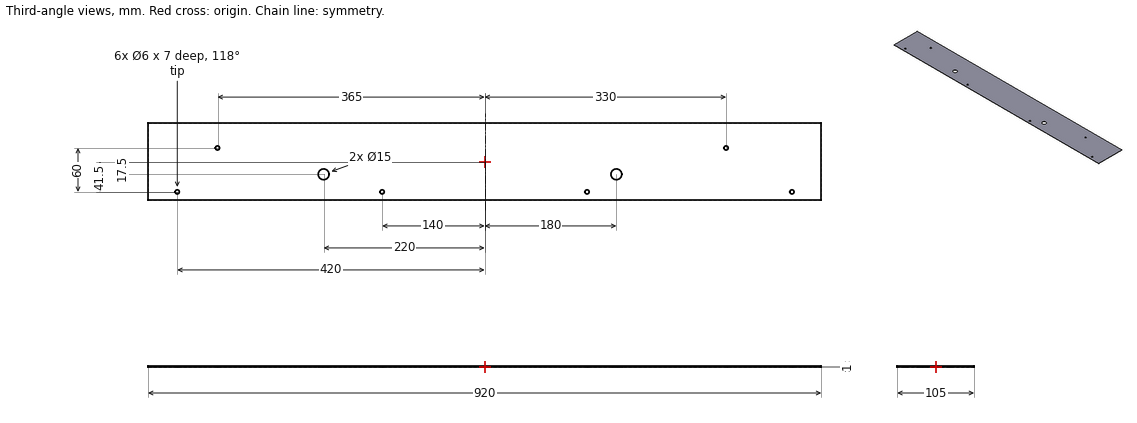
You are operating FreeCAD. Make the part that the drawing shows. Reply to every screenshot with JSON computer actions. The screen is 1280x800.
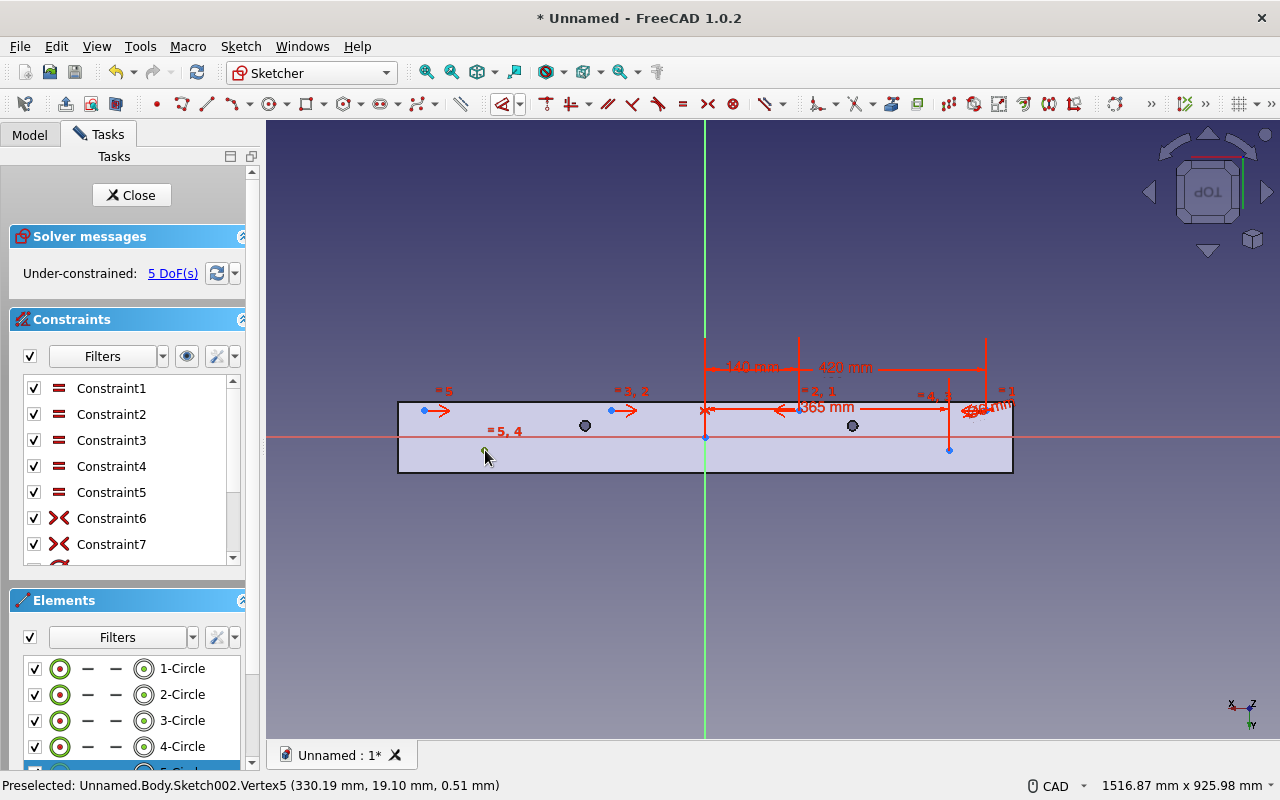
{"action": "left_click", "coordinate": [520, 104]}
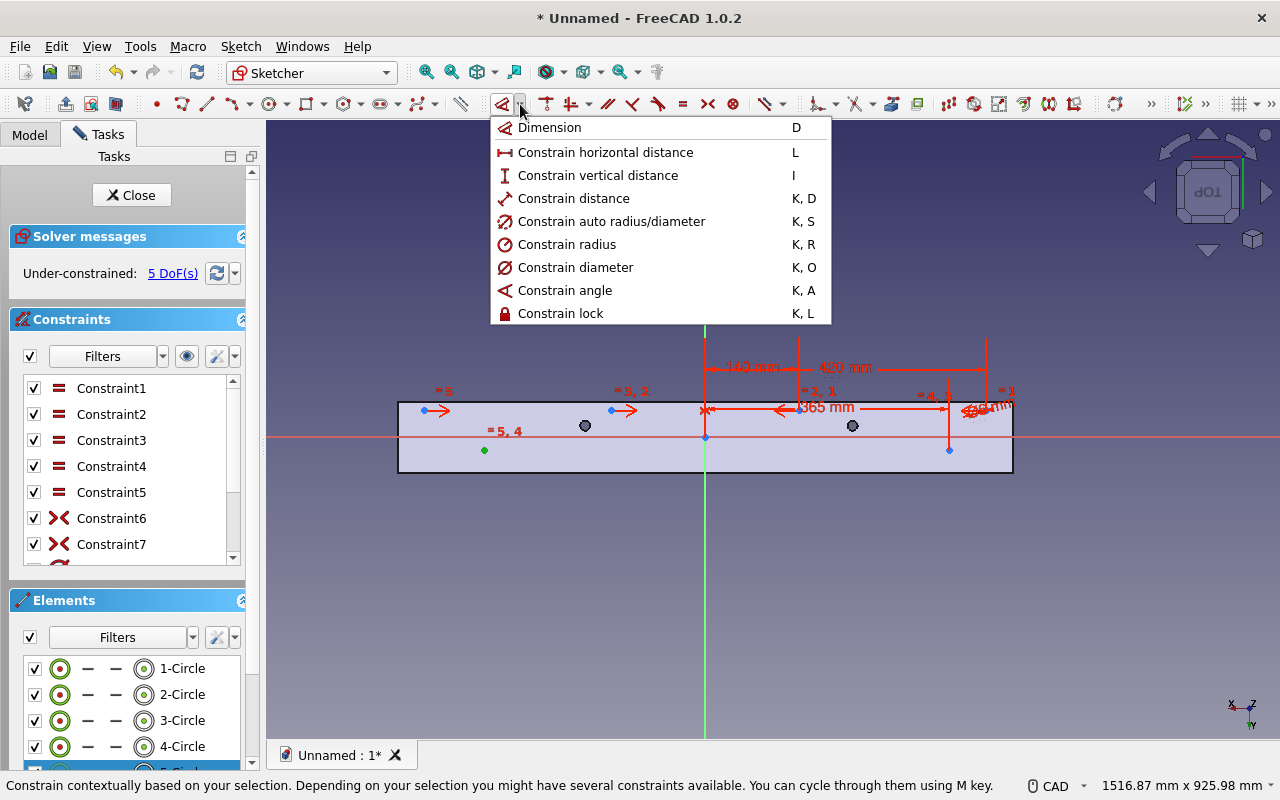
{"action": "left_click", "coordinate": [661, 152]}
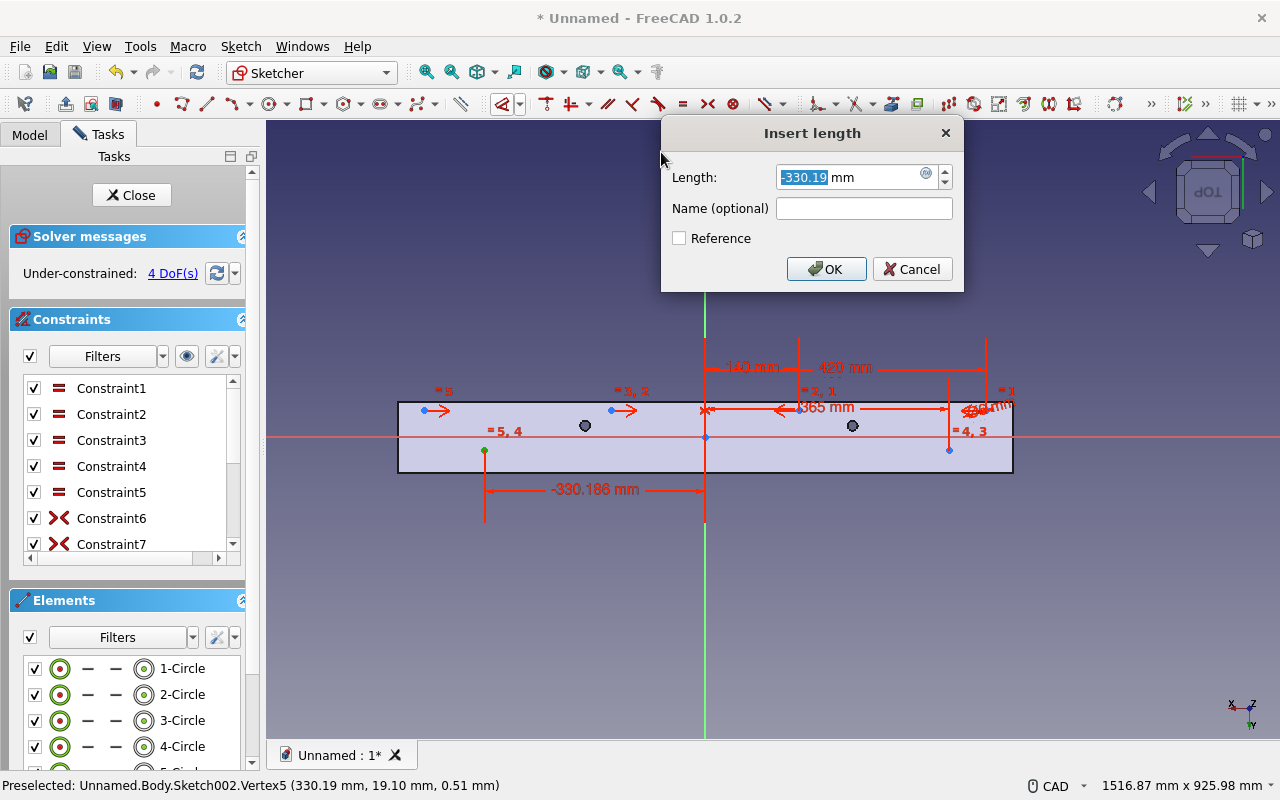
{"action": "type", "text": "-330"}
{"action": "key", "text": "Return"}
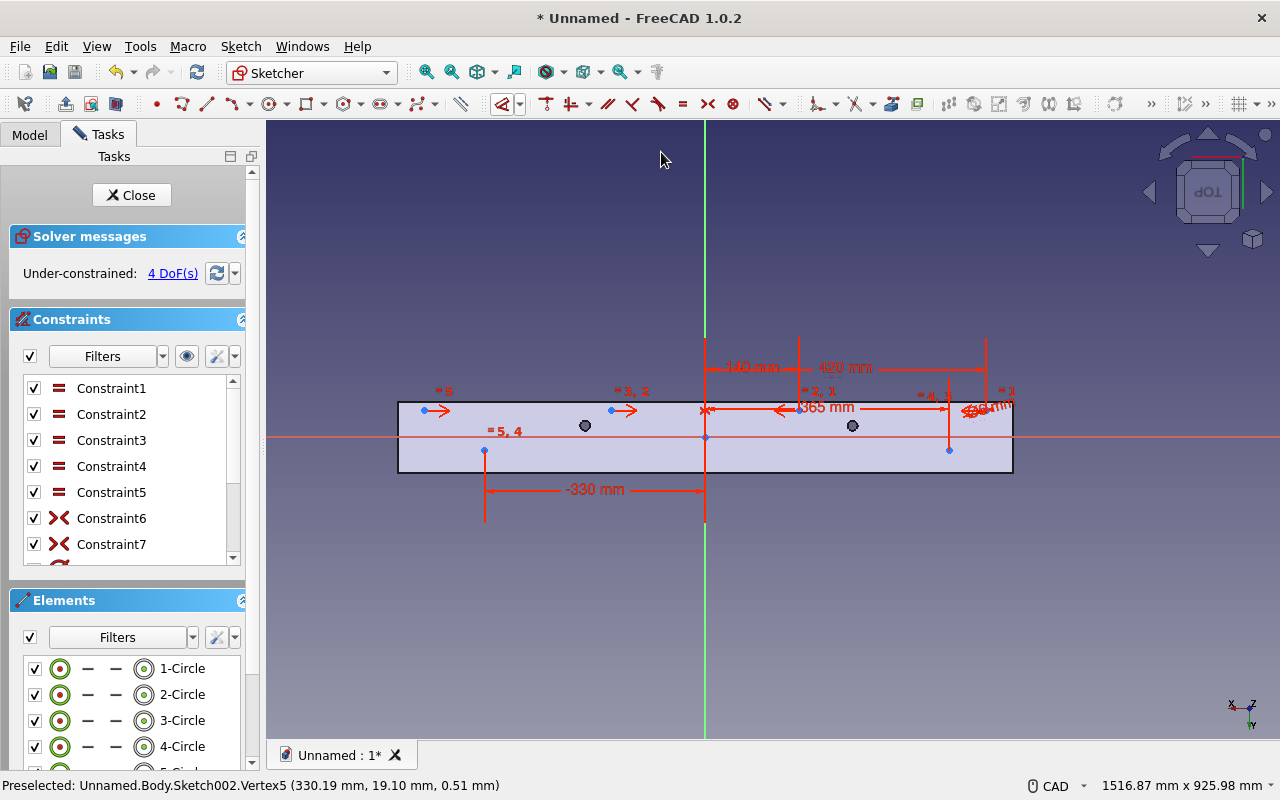
{"action": "left_click", "coordinate": [986, 411]}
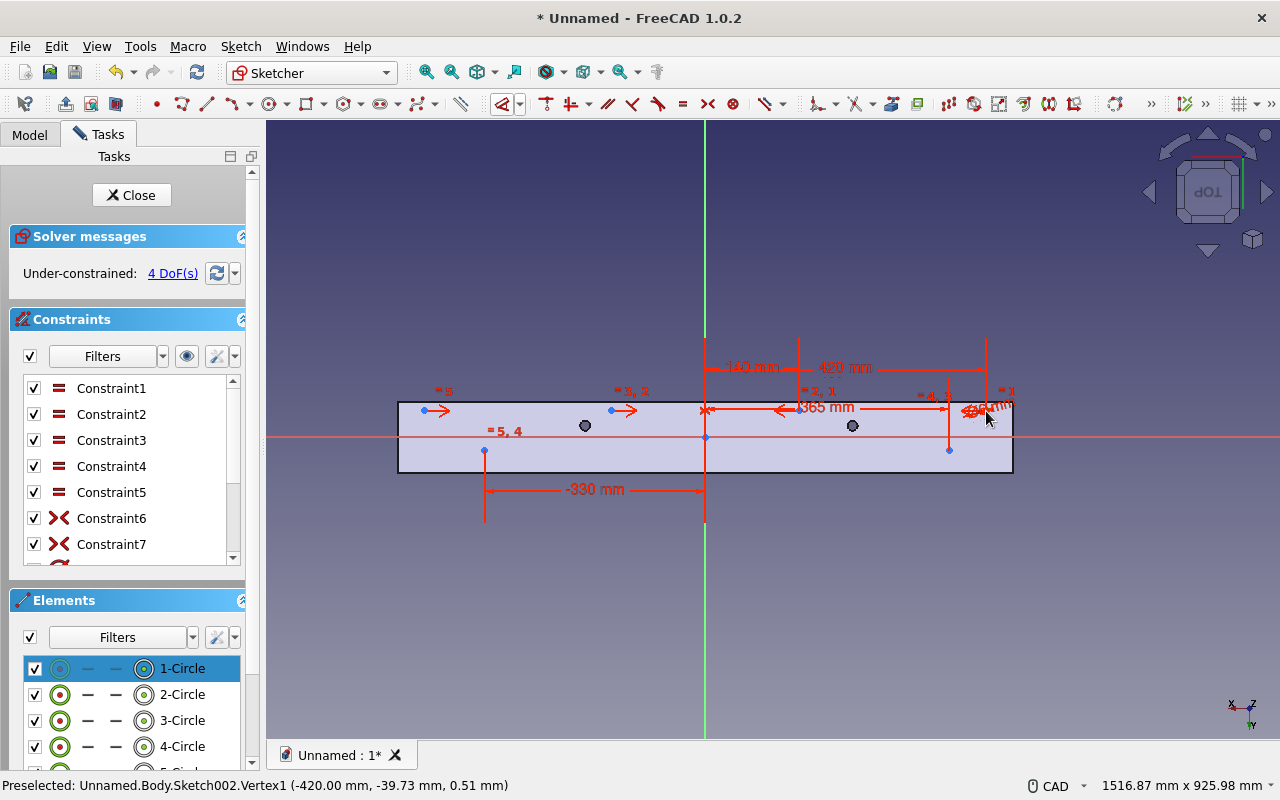
{"action": "left_click", "coordinate": [949, 450]}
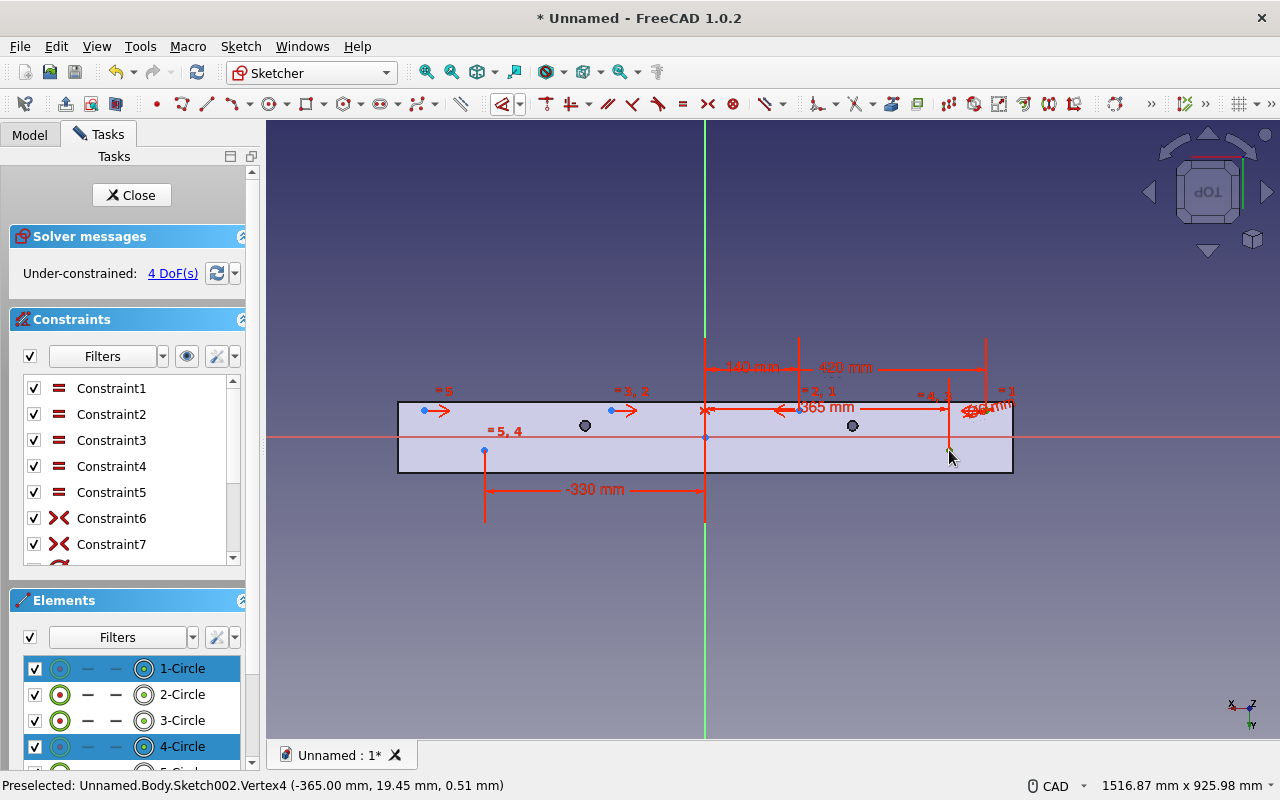
{"action": "key", "text": "i"}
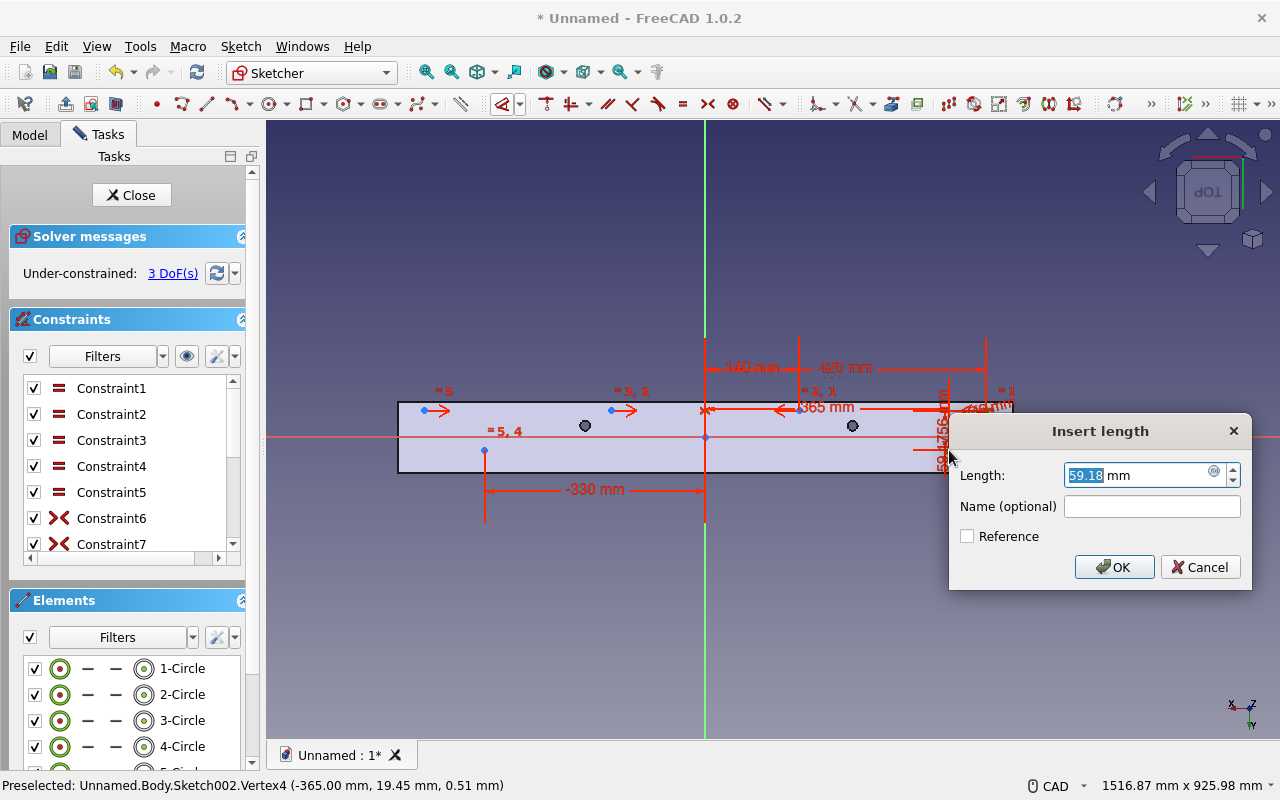
{"action": "type", "text": "60"}
{"action": "key", "text": "Return"}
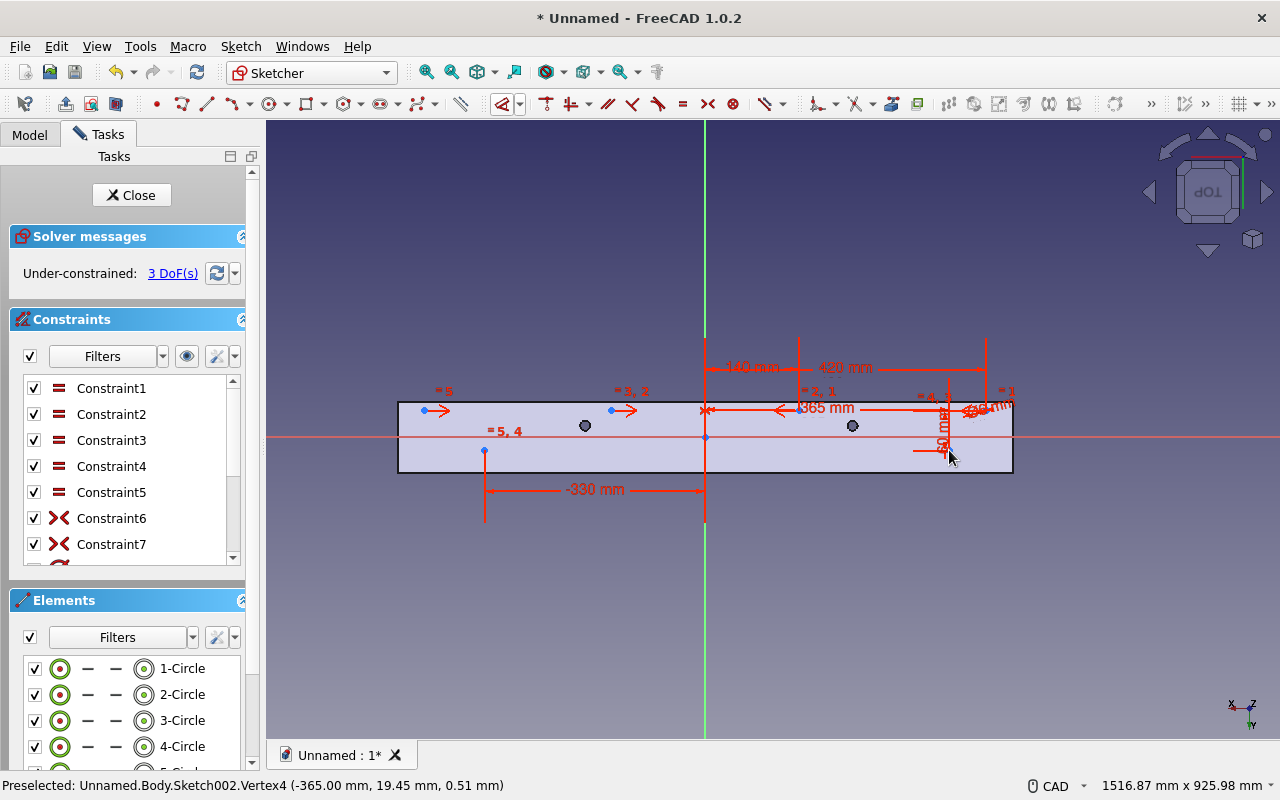
{"action": "left_click", "coordinate": [799, 411]}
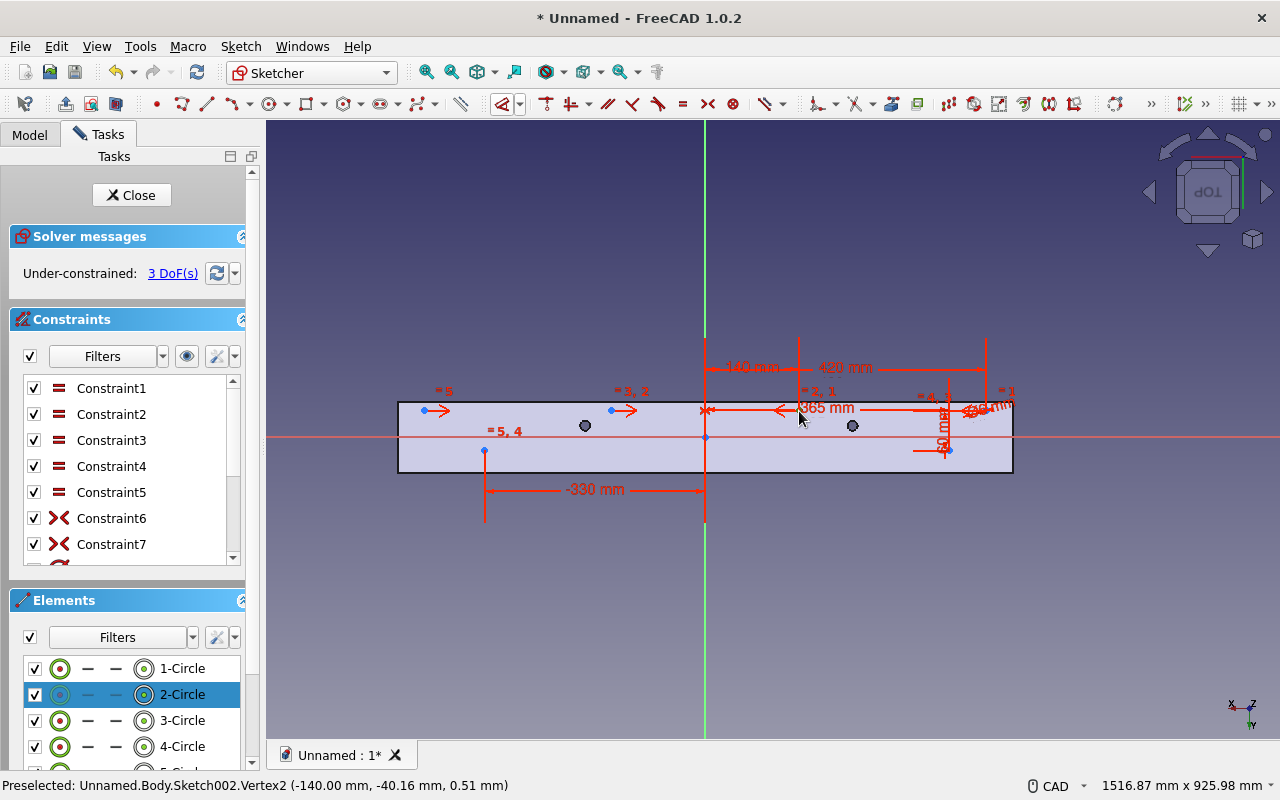
{"action": "left_click", "coordinate": [949, 451]}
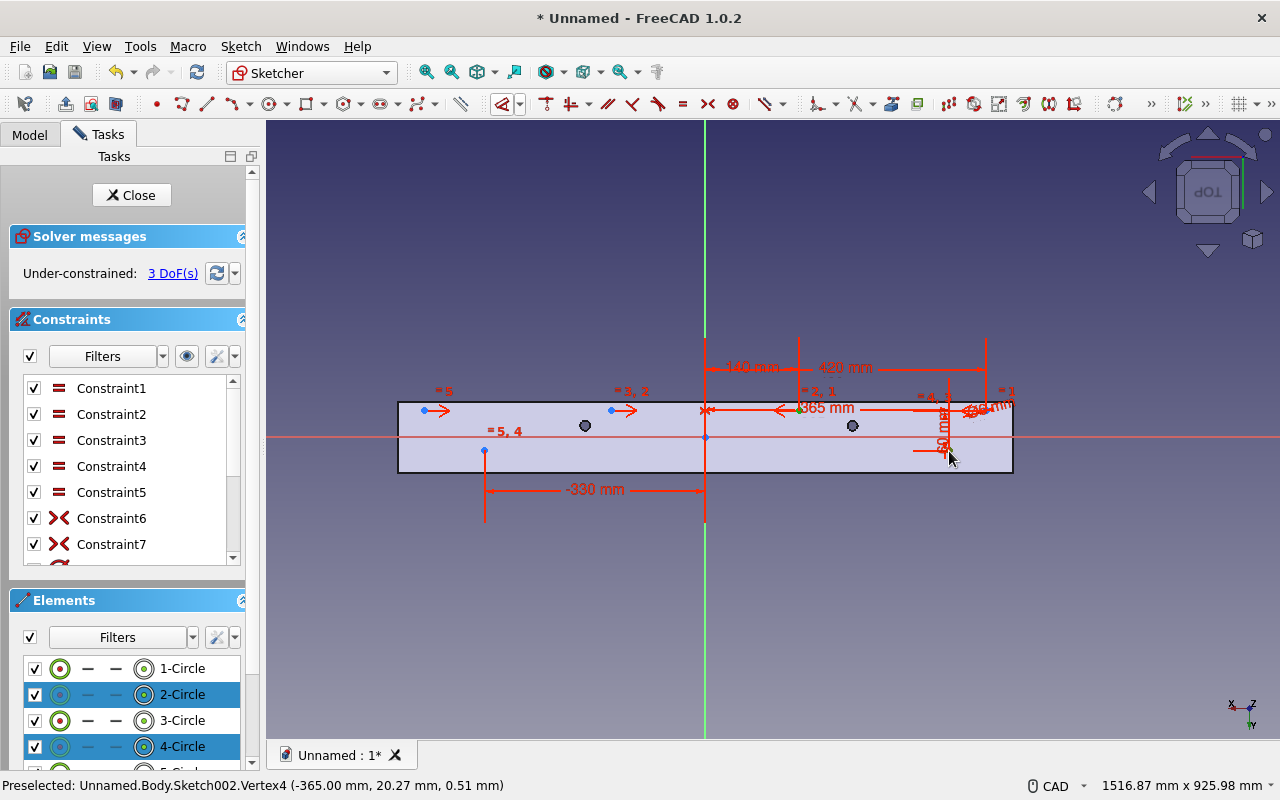
{"action": "left_click", "coordinate": [520, 104]}